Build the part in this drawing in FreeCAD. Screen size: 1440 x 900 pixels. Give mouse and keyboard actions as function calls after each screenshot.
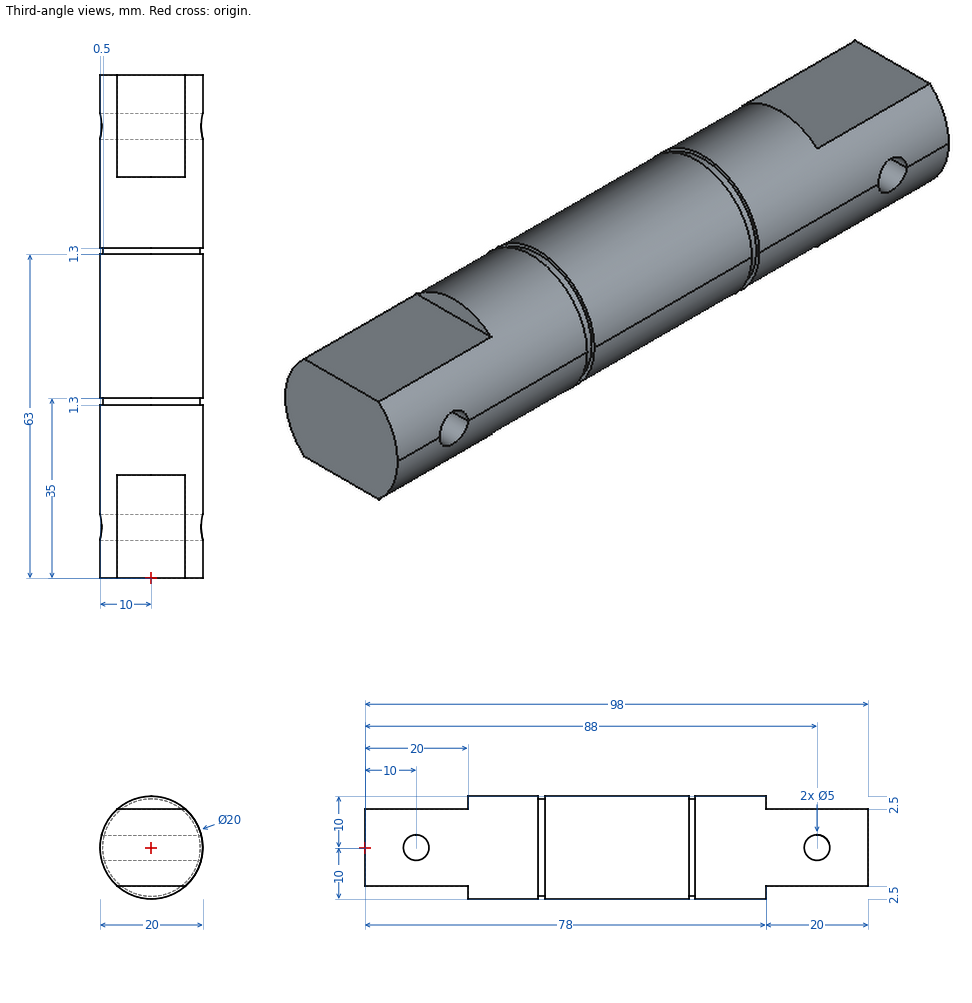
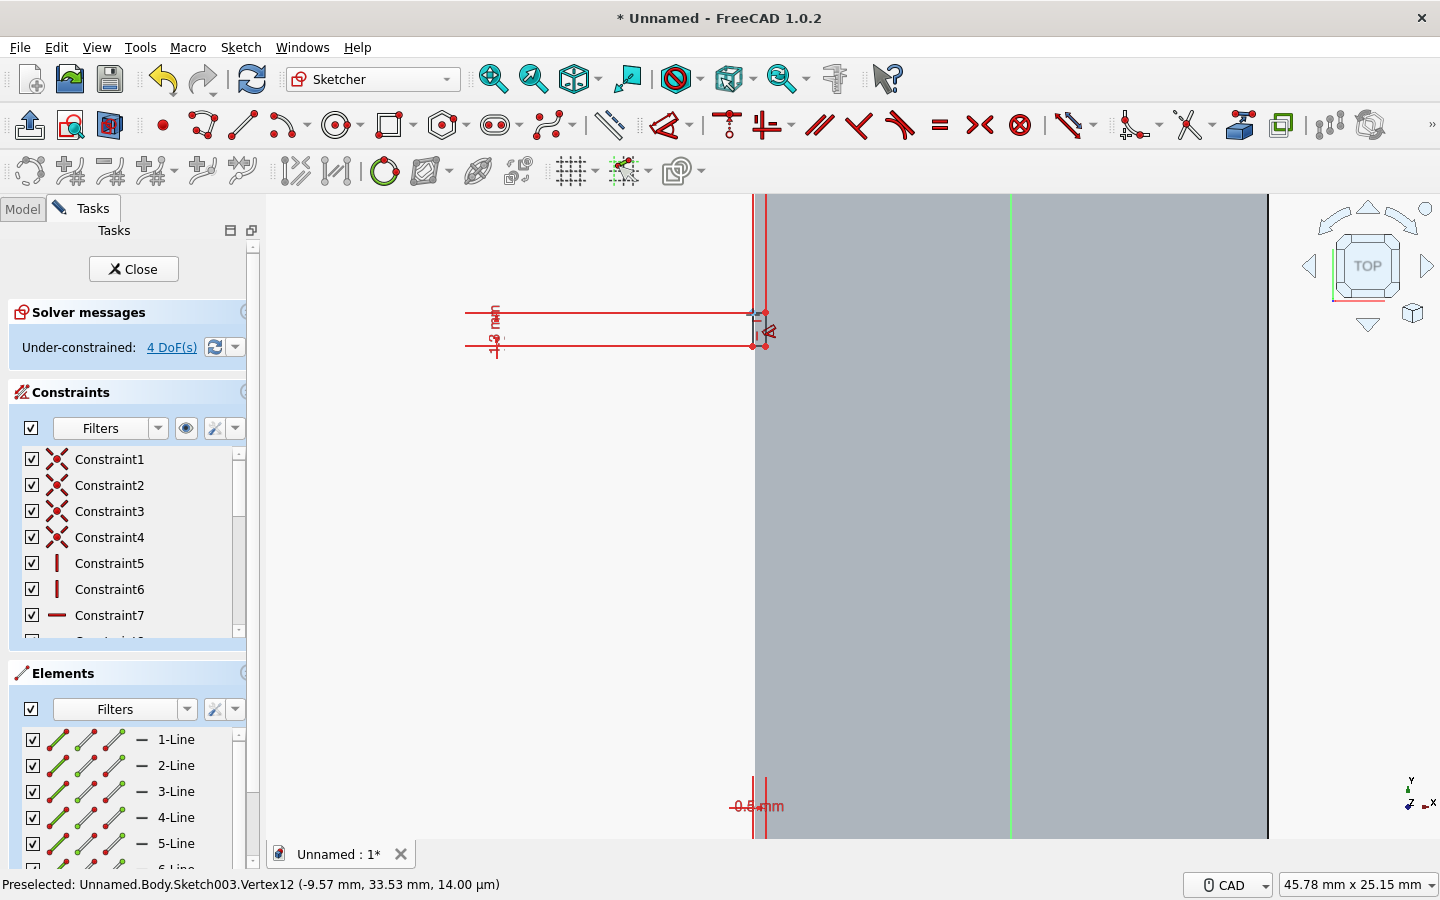
click(753, 313)
click(882, 279)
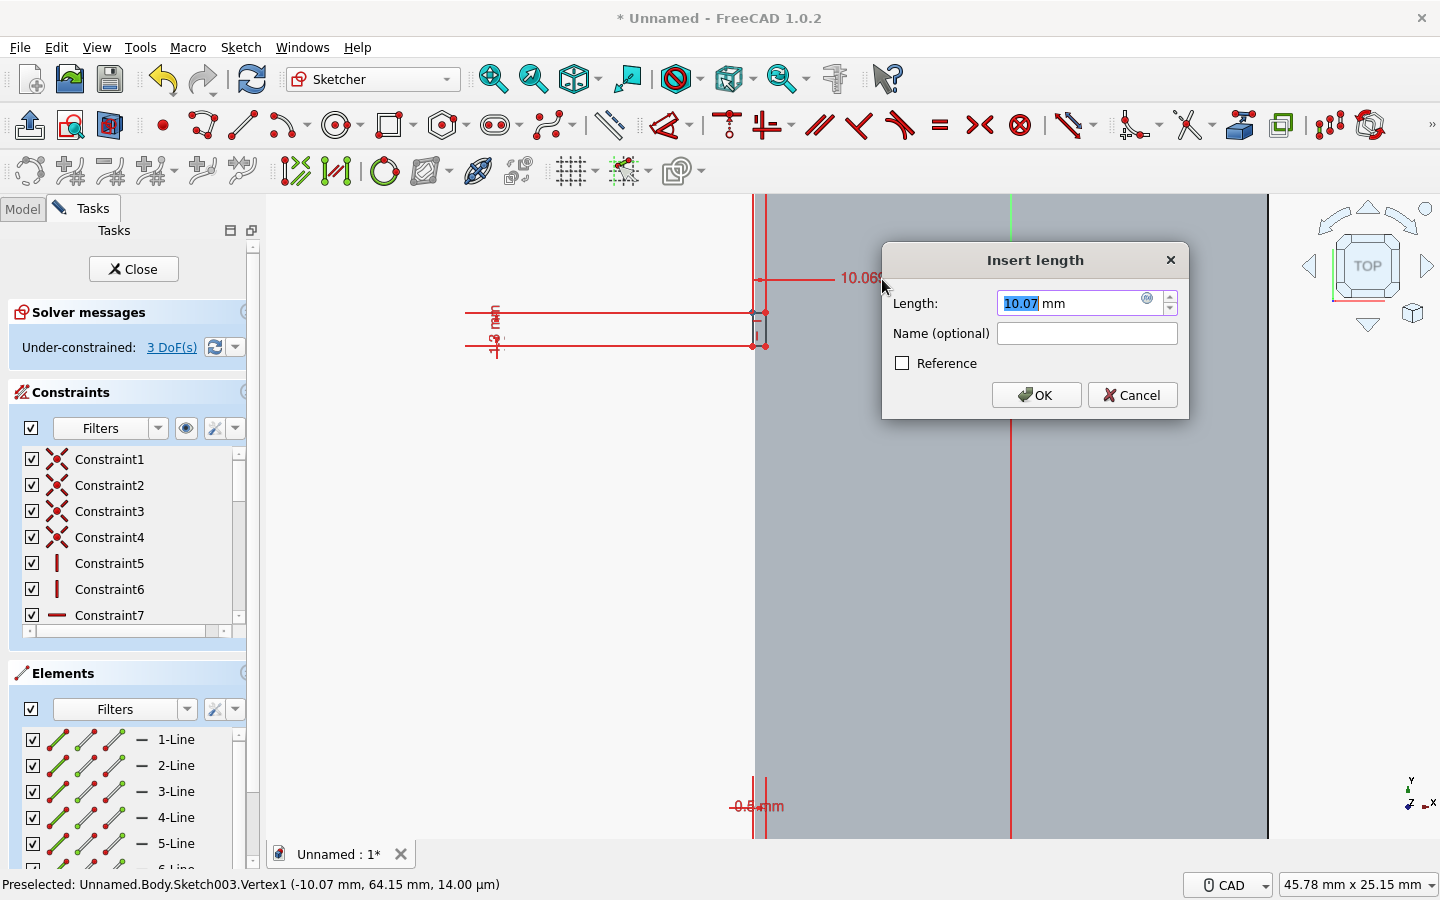
text(10)
key(Return)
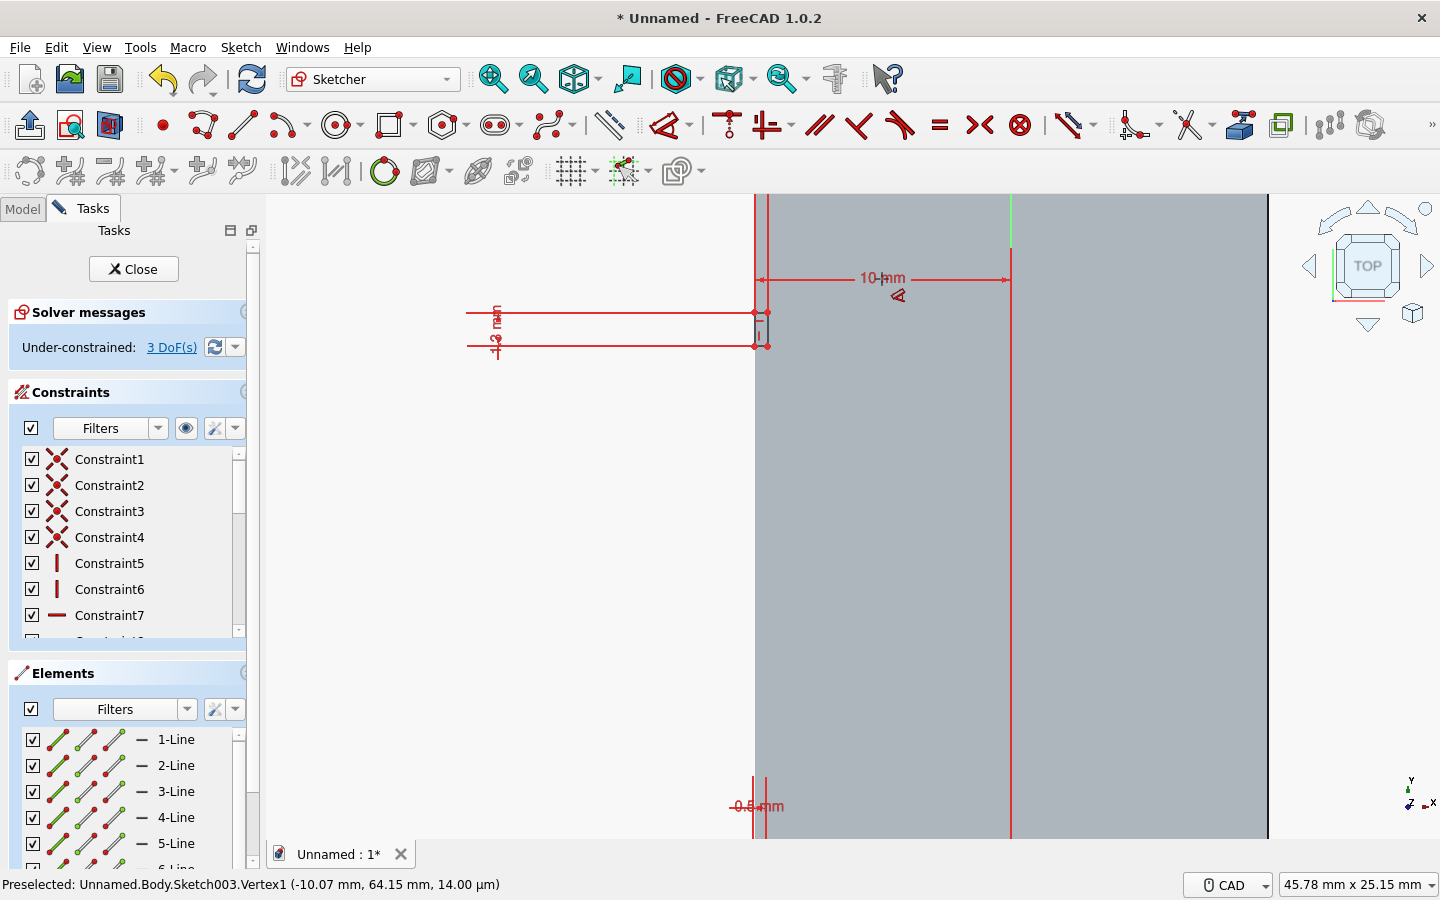
click(755, 346)
click(1045, 579)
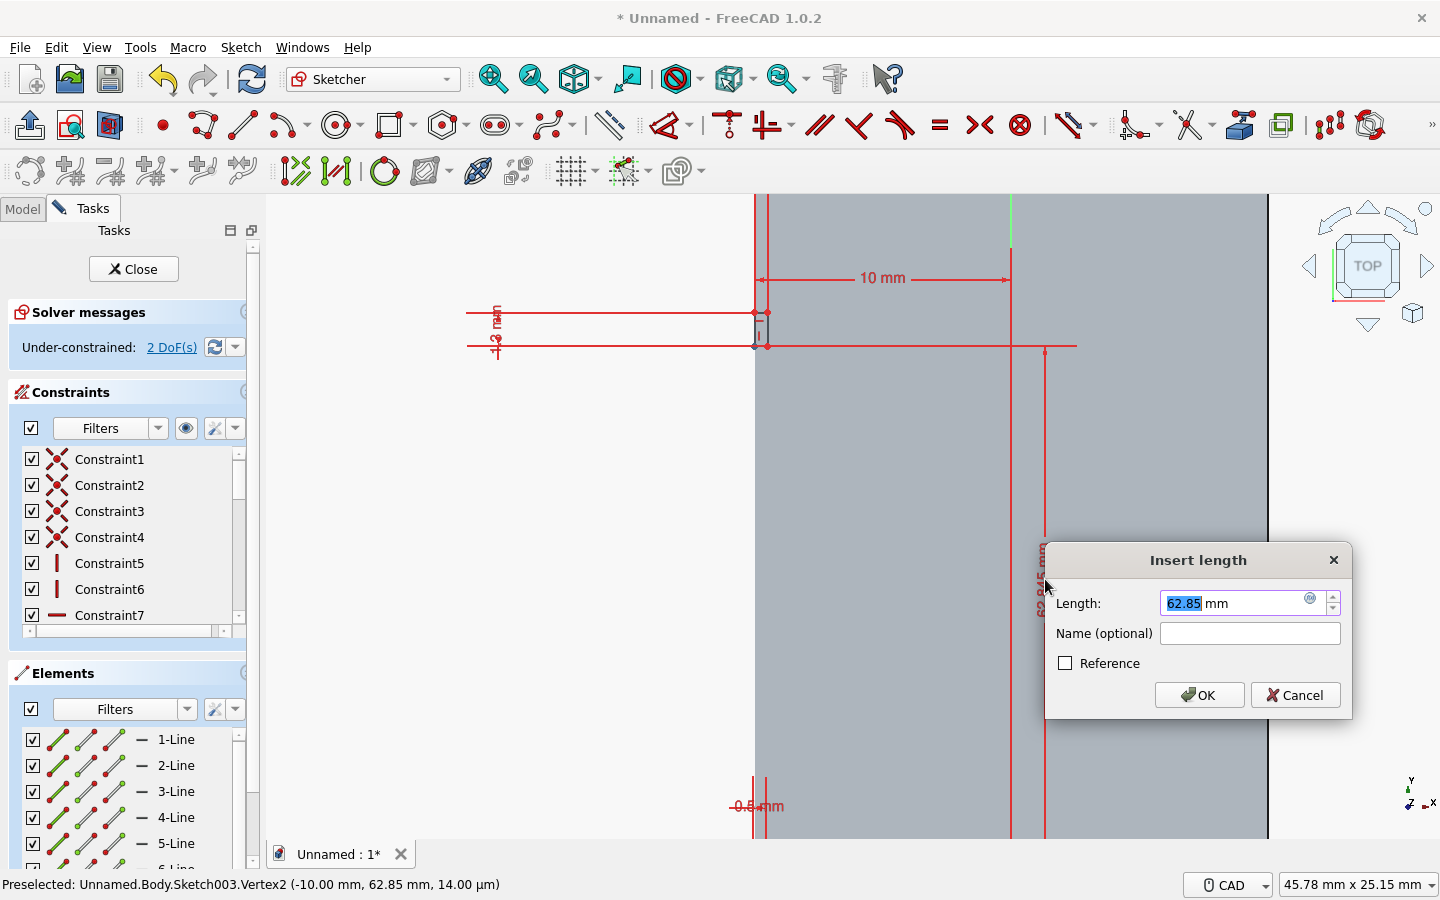
text(63)
key(Return)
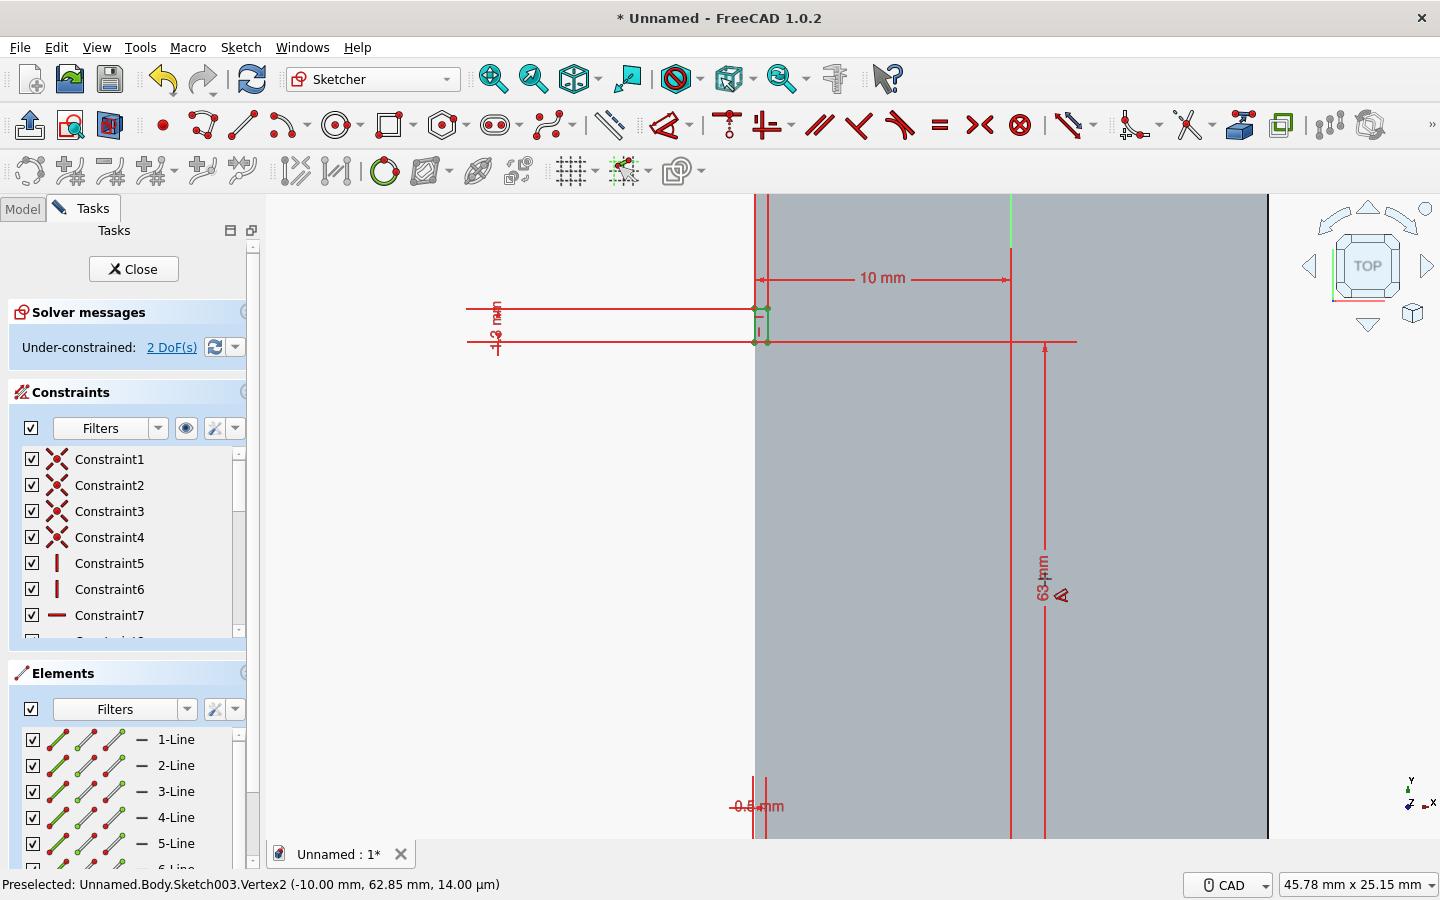
scroll(752, 315, down, 7)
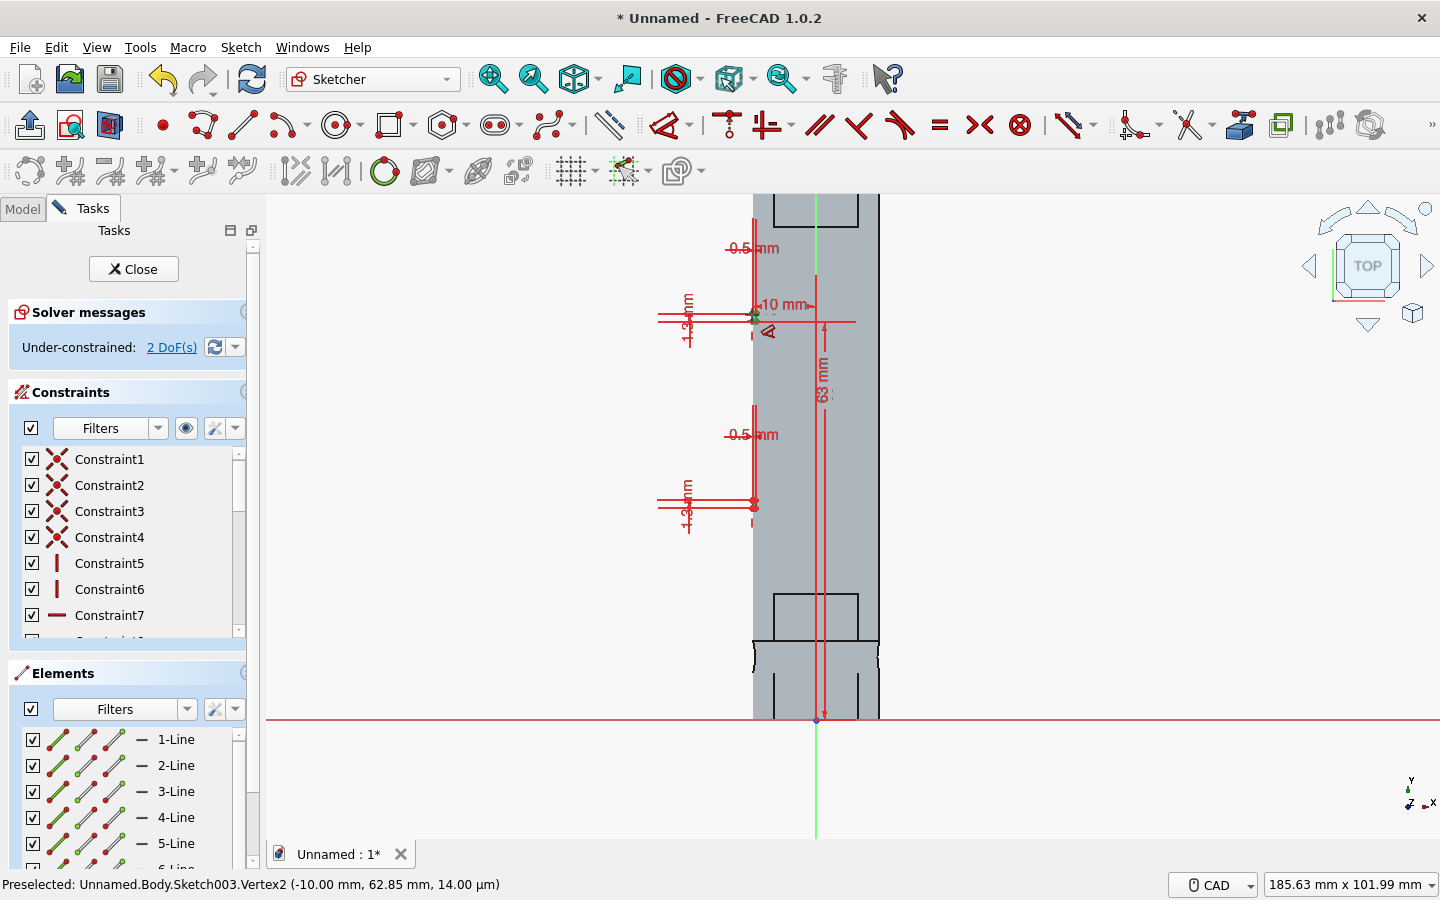
scroll(753, 500, up, 7)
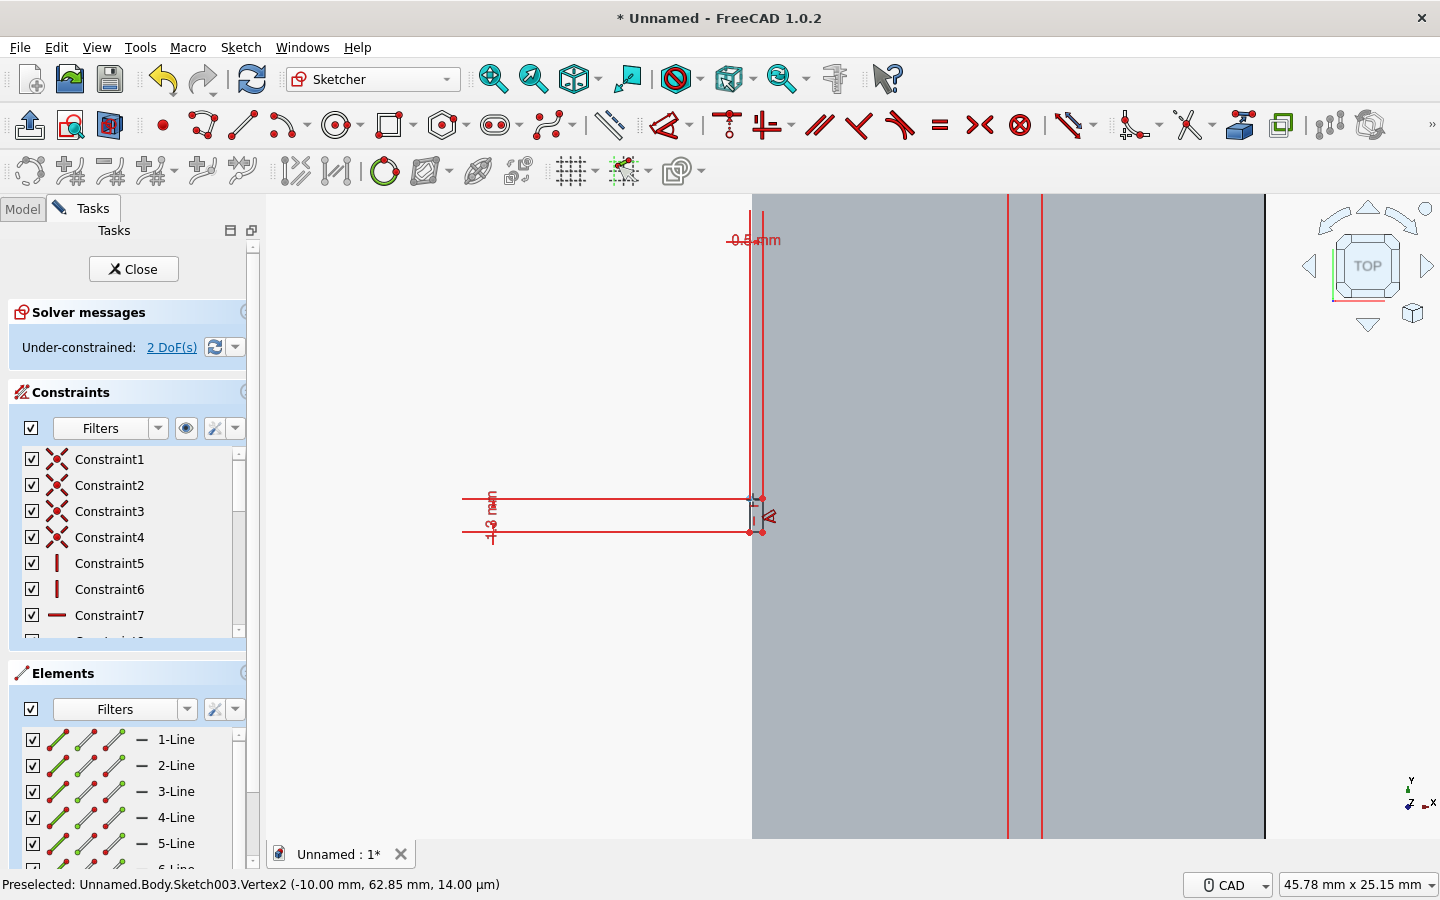
click(750, 499)
click(879, 465)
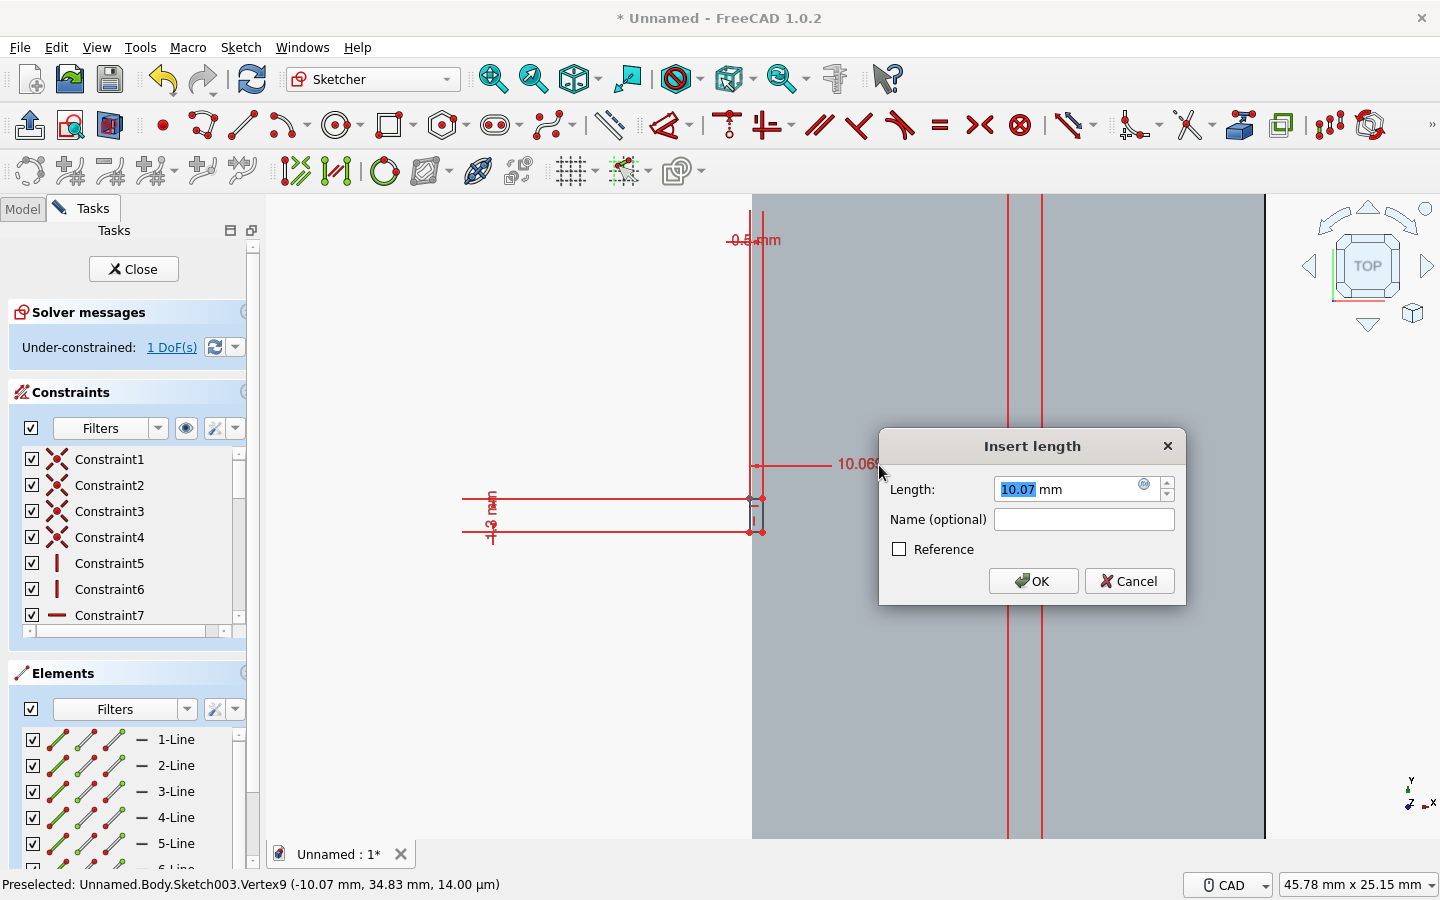
text(10)
key(Return)